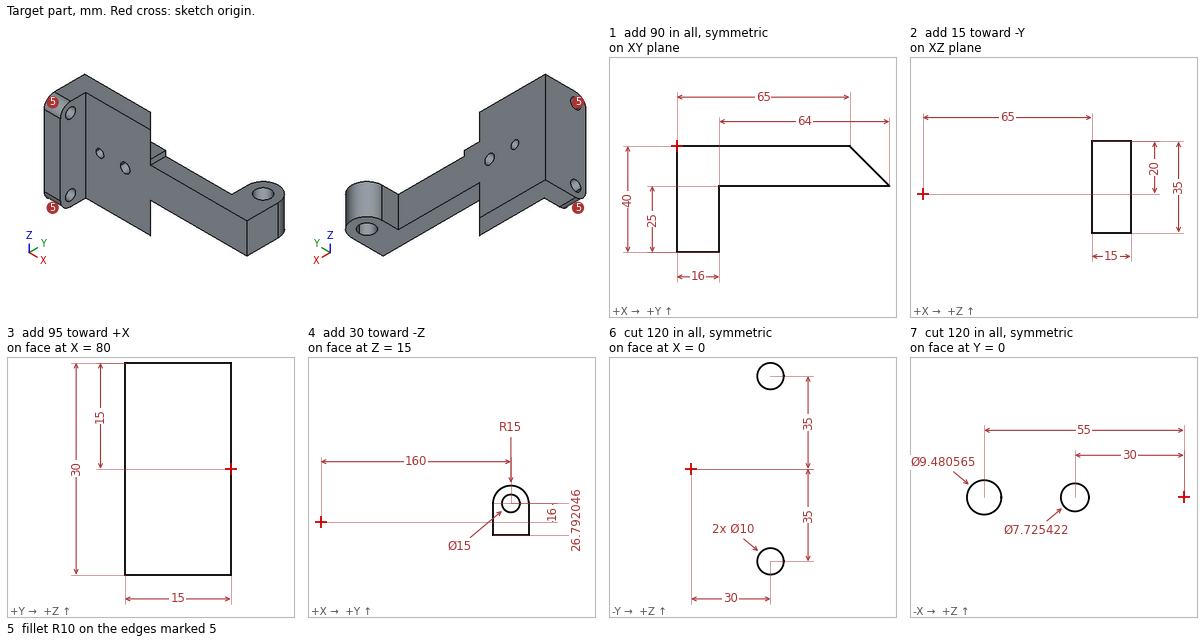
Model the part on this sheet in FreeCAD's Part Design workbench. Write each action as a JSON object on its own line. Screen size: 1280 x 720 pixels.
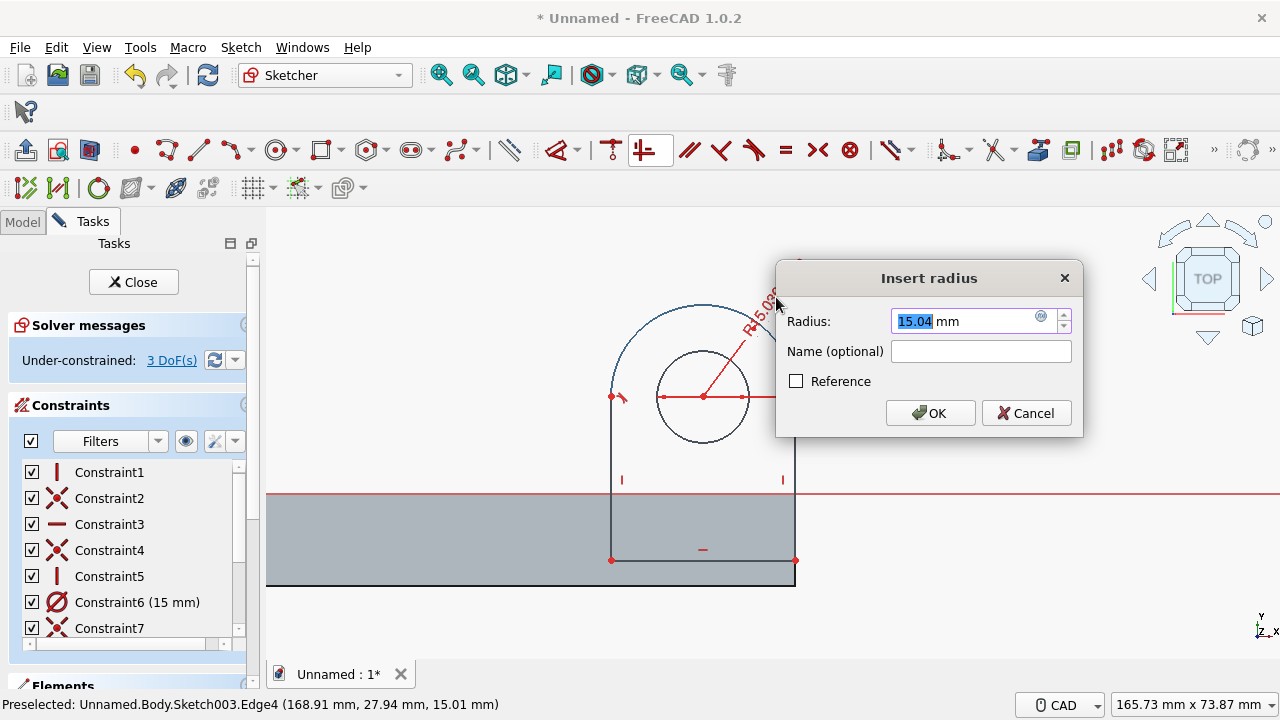
{"action": "type", "text": "15"}
{"action": "key", "text": "Return"}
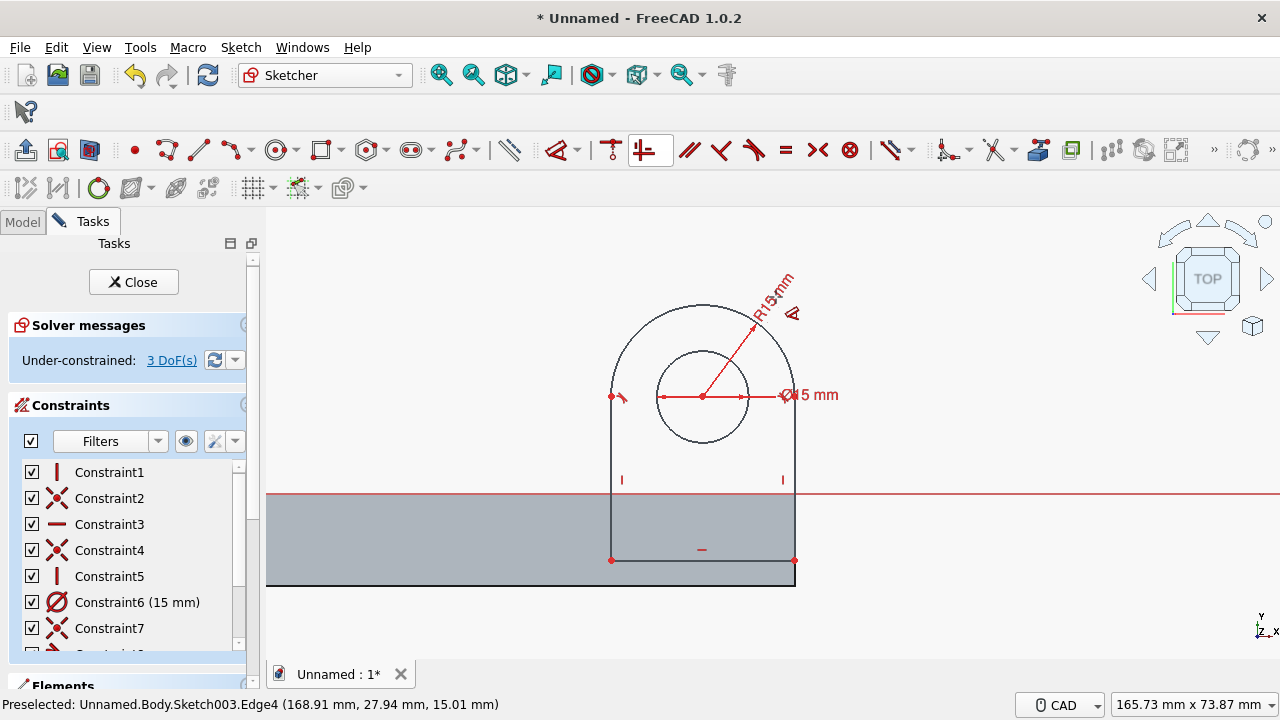
{"action": "left_click", "coordinate": [703, 397]}
{"action": "left_click", "coordinate": [737, 446]}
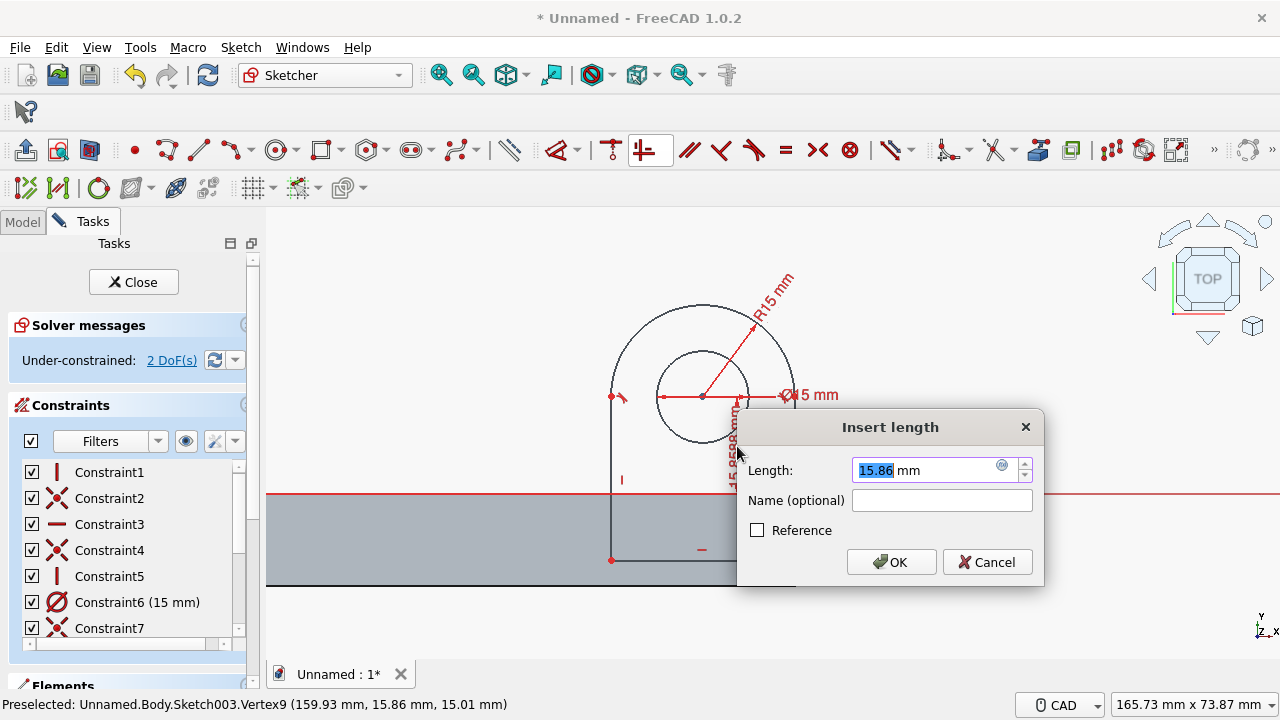
{"action": "type", "text": "16"}
{"action": "key", "text": "Return"}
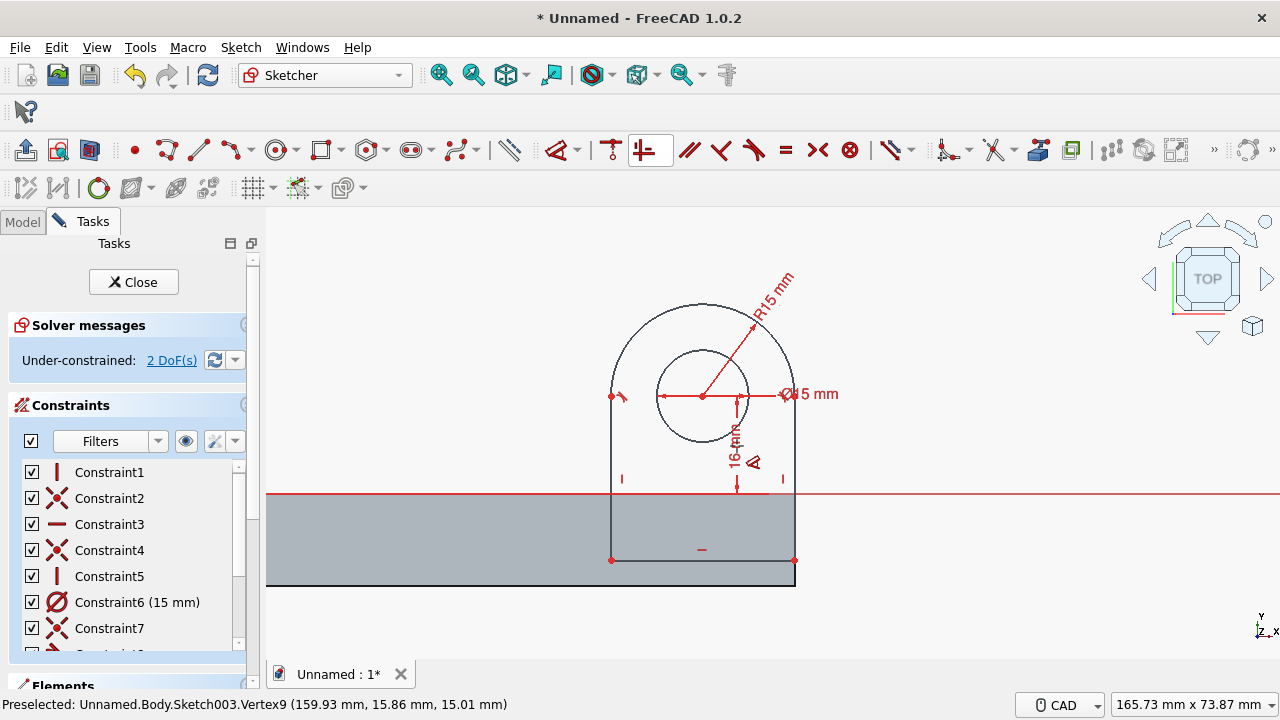
{"action": "left_click", "coordinate": [703, 396]}
{"action": "left_click", "coordinate": [498, 528]}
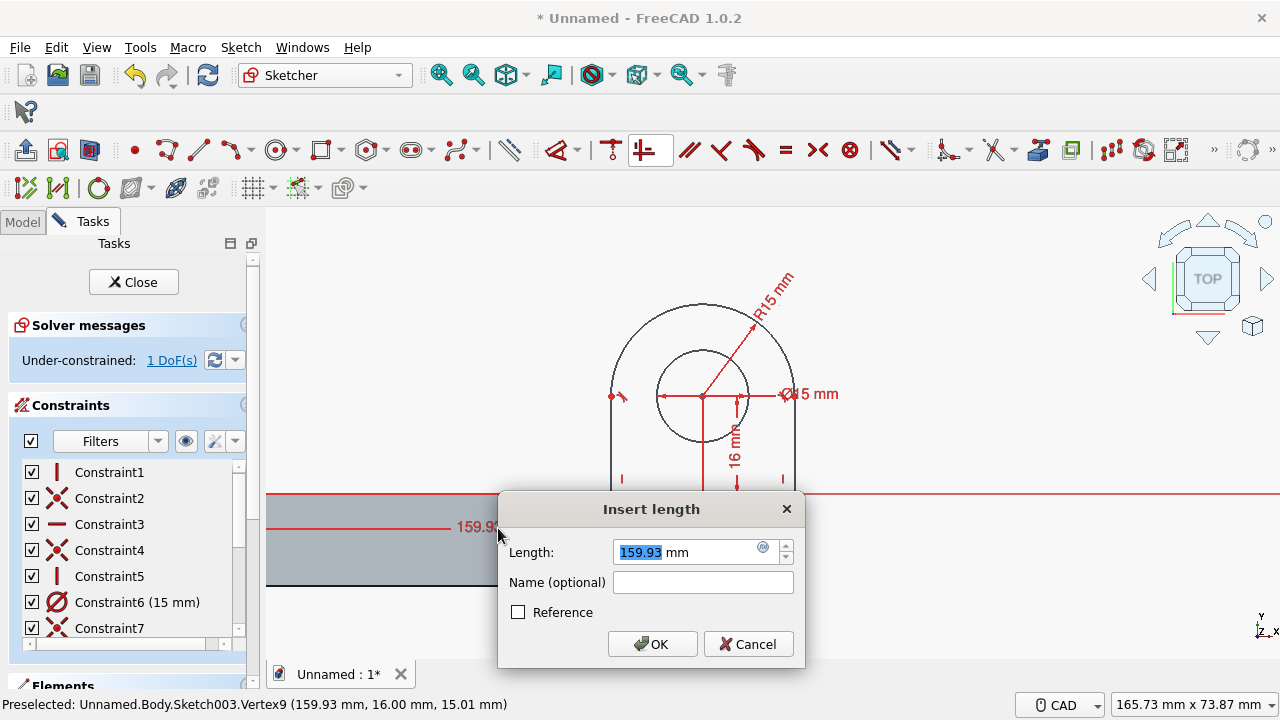
{"action": "type", "text": "160"}
{"action": "key", "text": "Return"}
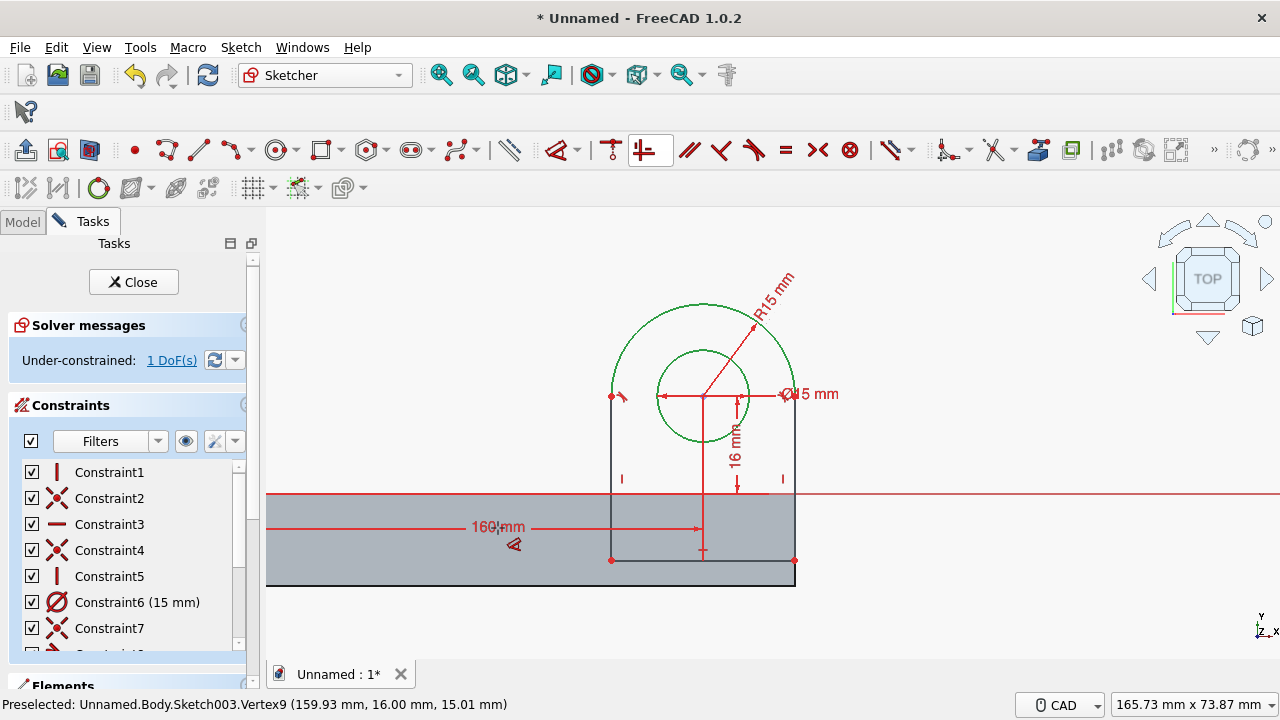
{"action": "left_click", "coordinate": [611, 446]}
{"action": "left_click", "coordinate": [577, 479]}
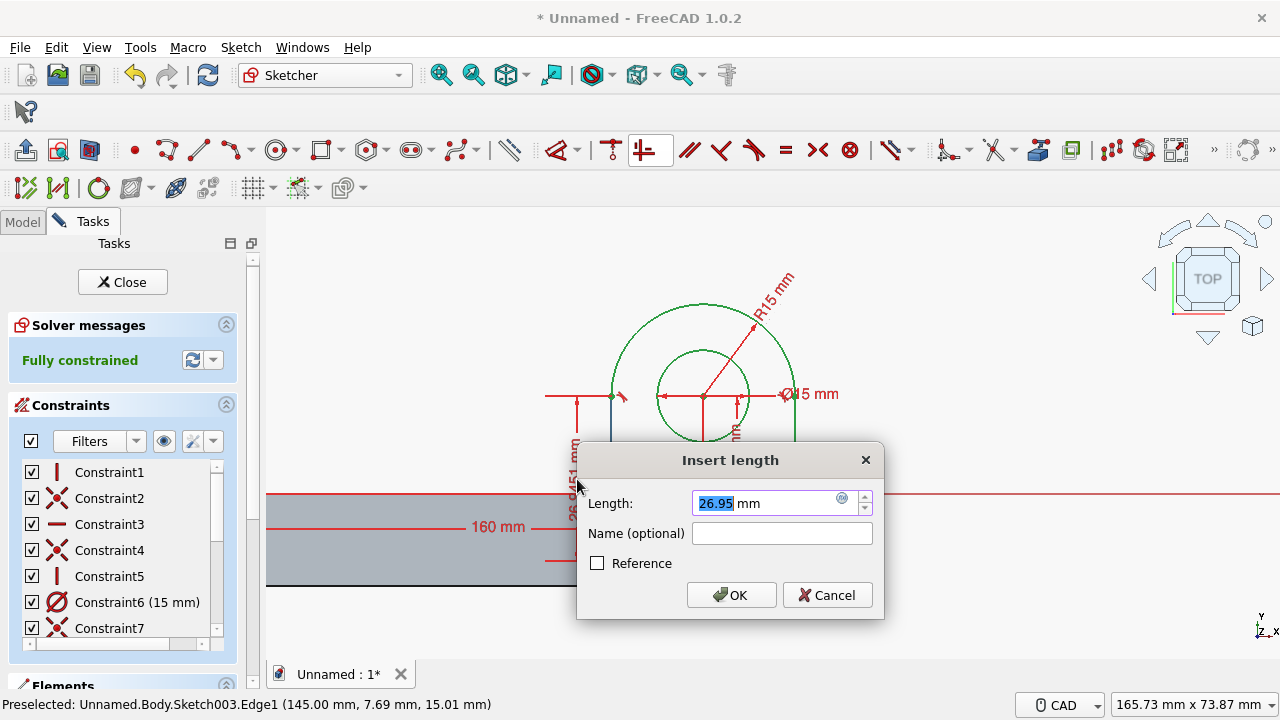
{"action": "type", "text": "26.792046"}
{"action": "key", "text": "Return"}
{"action": "key", "text": "Escape"}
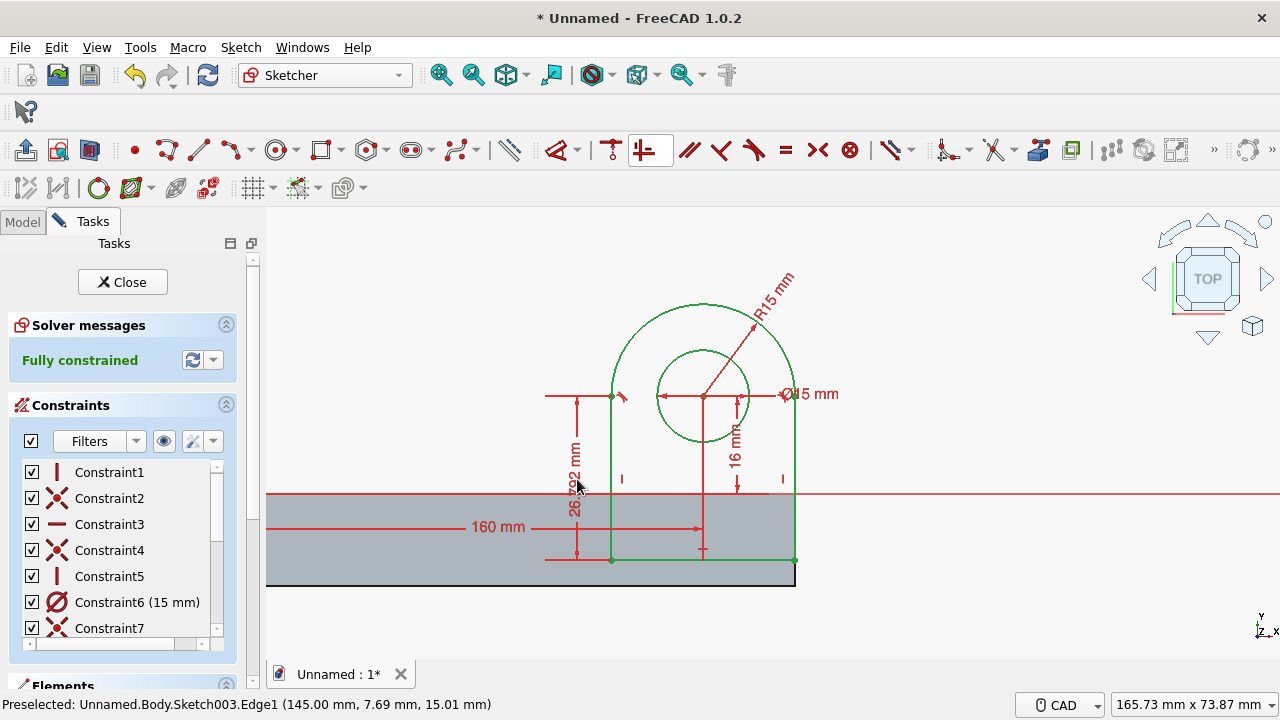
{"action": "left_click", "coordinate": [123, 282]}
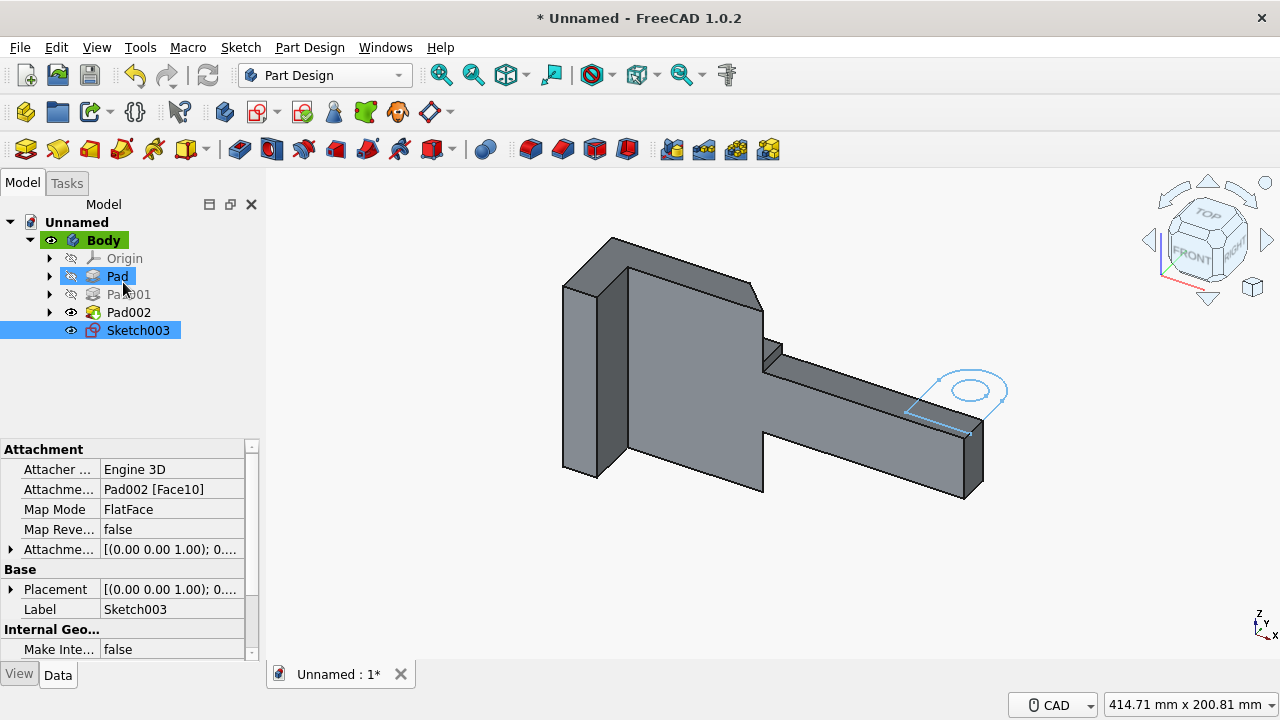
{"action": "left_click", "coordinate": [26, 150]}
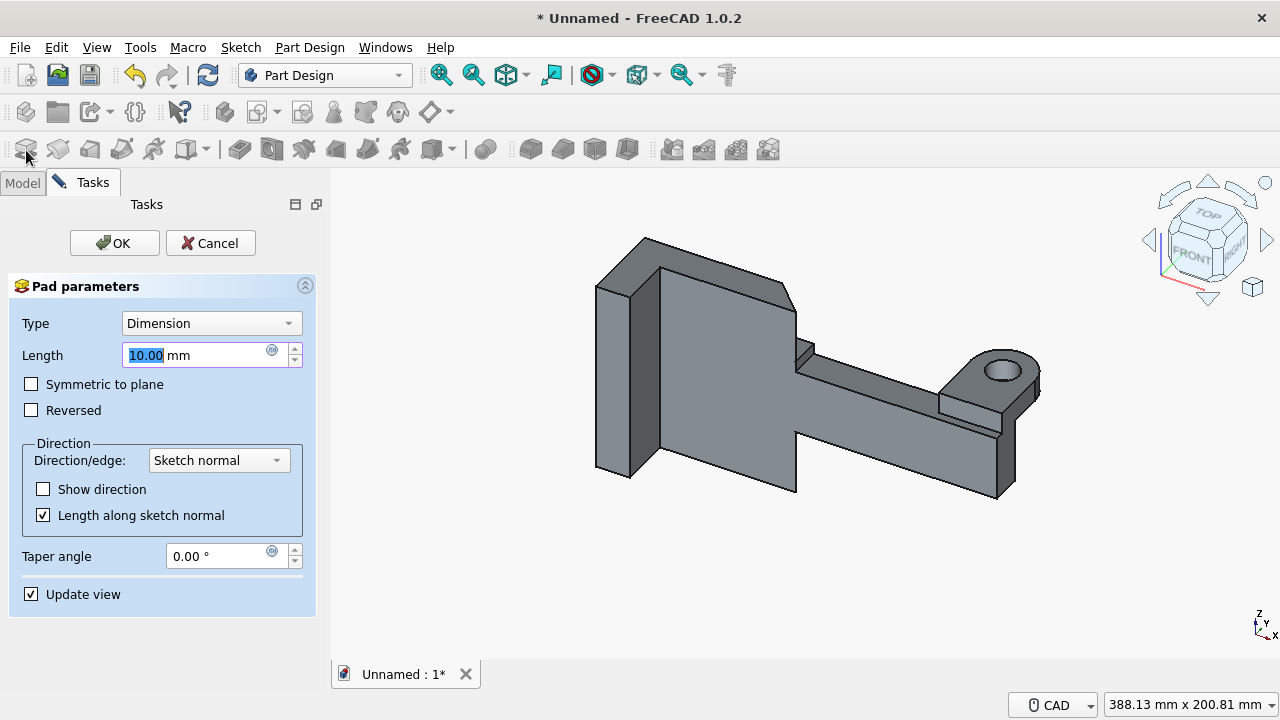
{"action": "type", "text": "30"}
{"action": "key", "text": "Tab"}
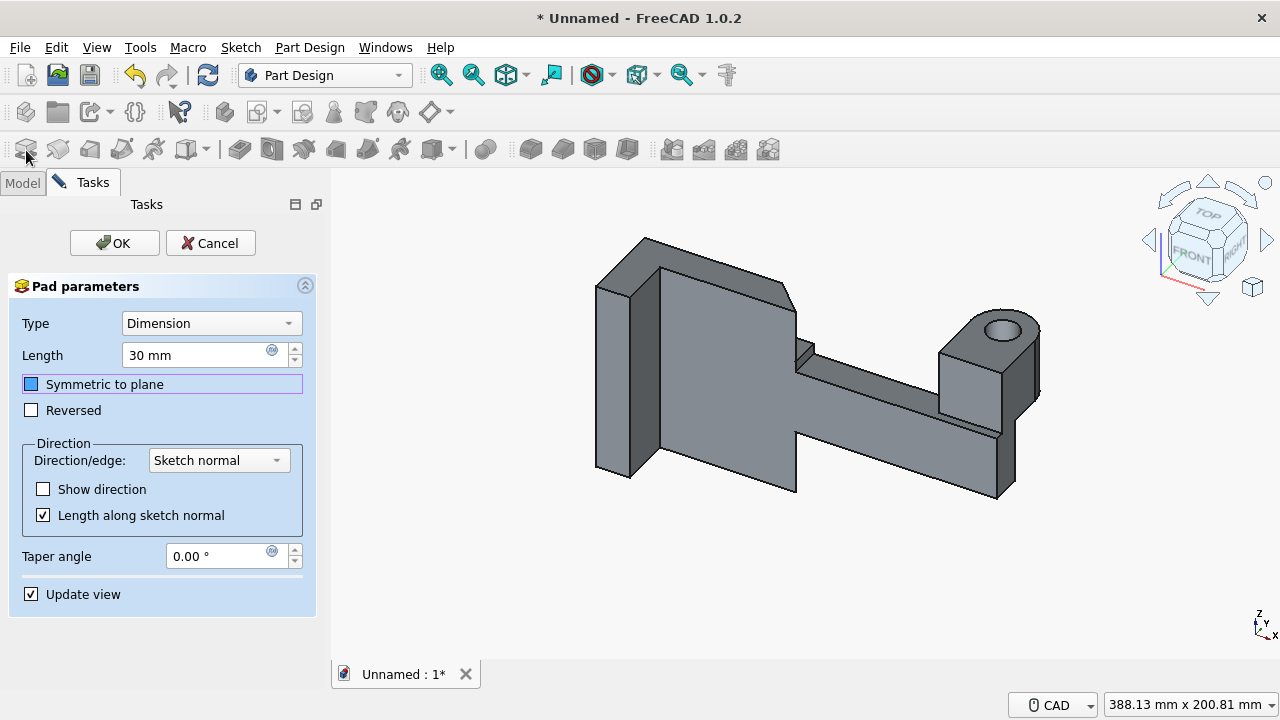
{"action": "left_click", "coordinate": [30, 410]}